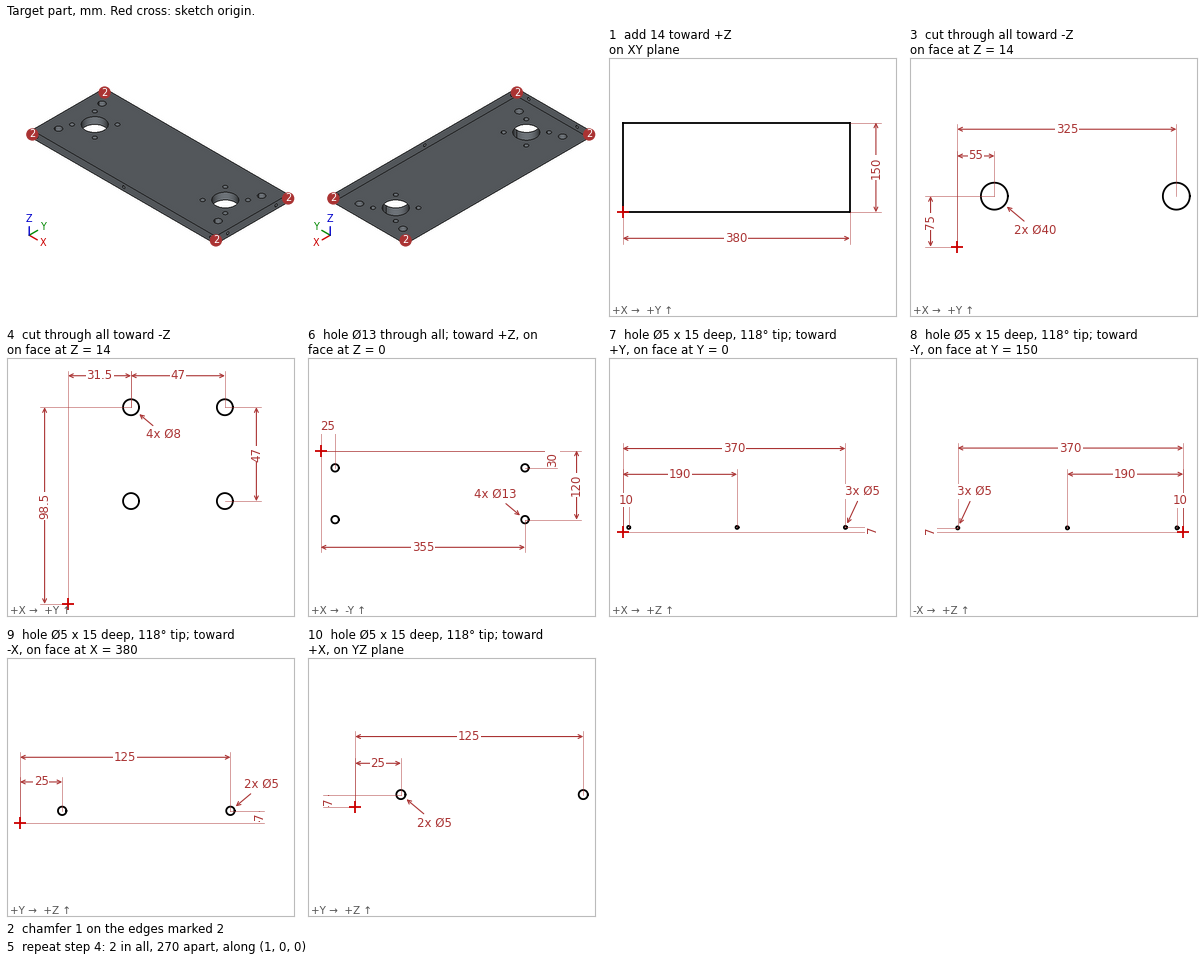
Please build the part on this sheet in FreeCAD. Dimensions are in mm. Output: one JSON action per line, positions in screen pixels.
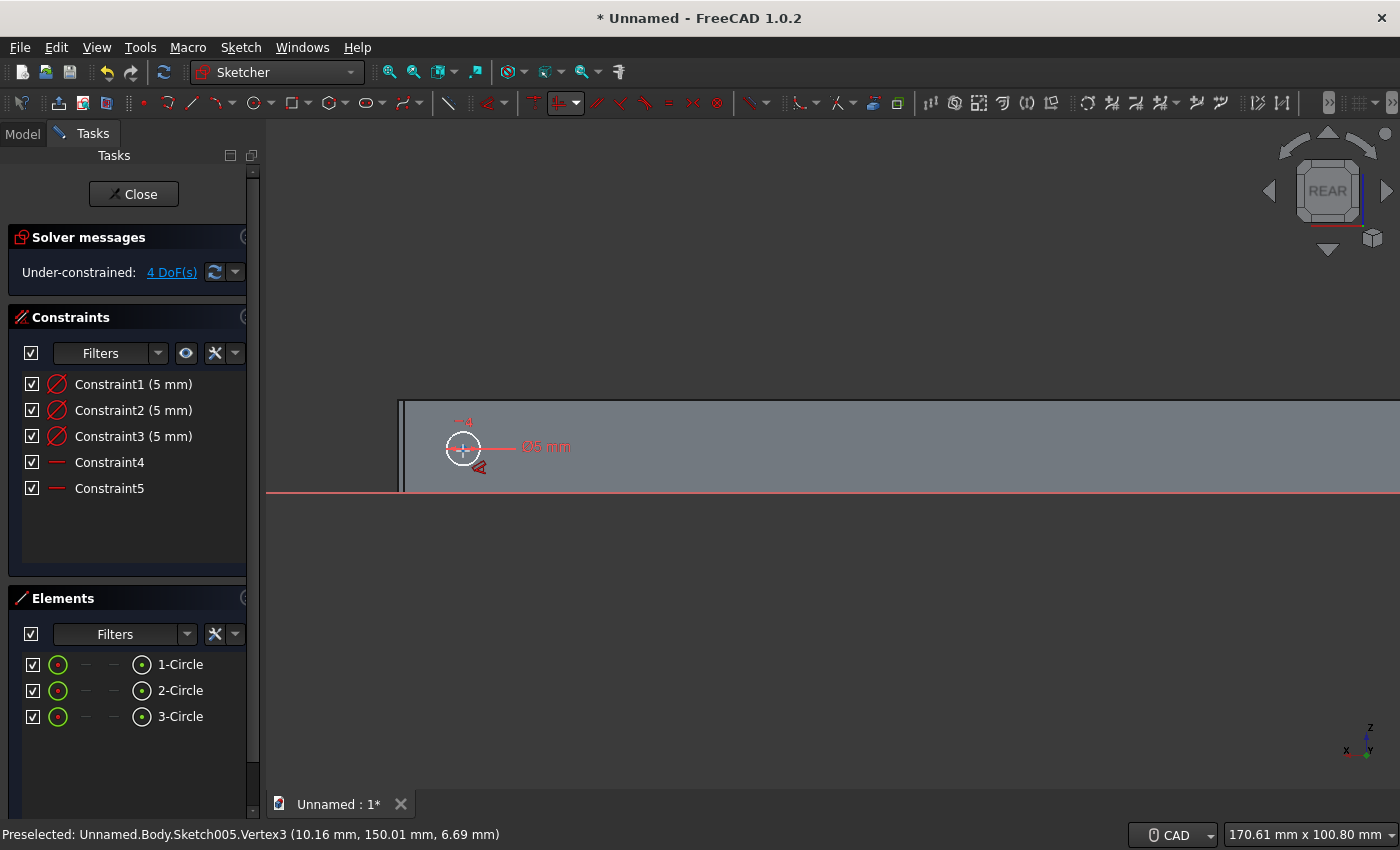
{"action": "left_click", "coordinate": [463, 449]}
{"action": "left_click", "coordinate": [429, 471]}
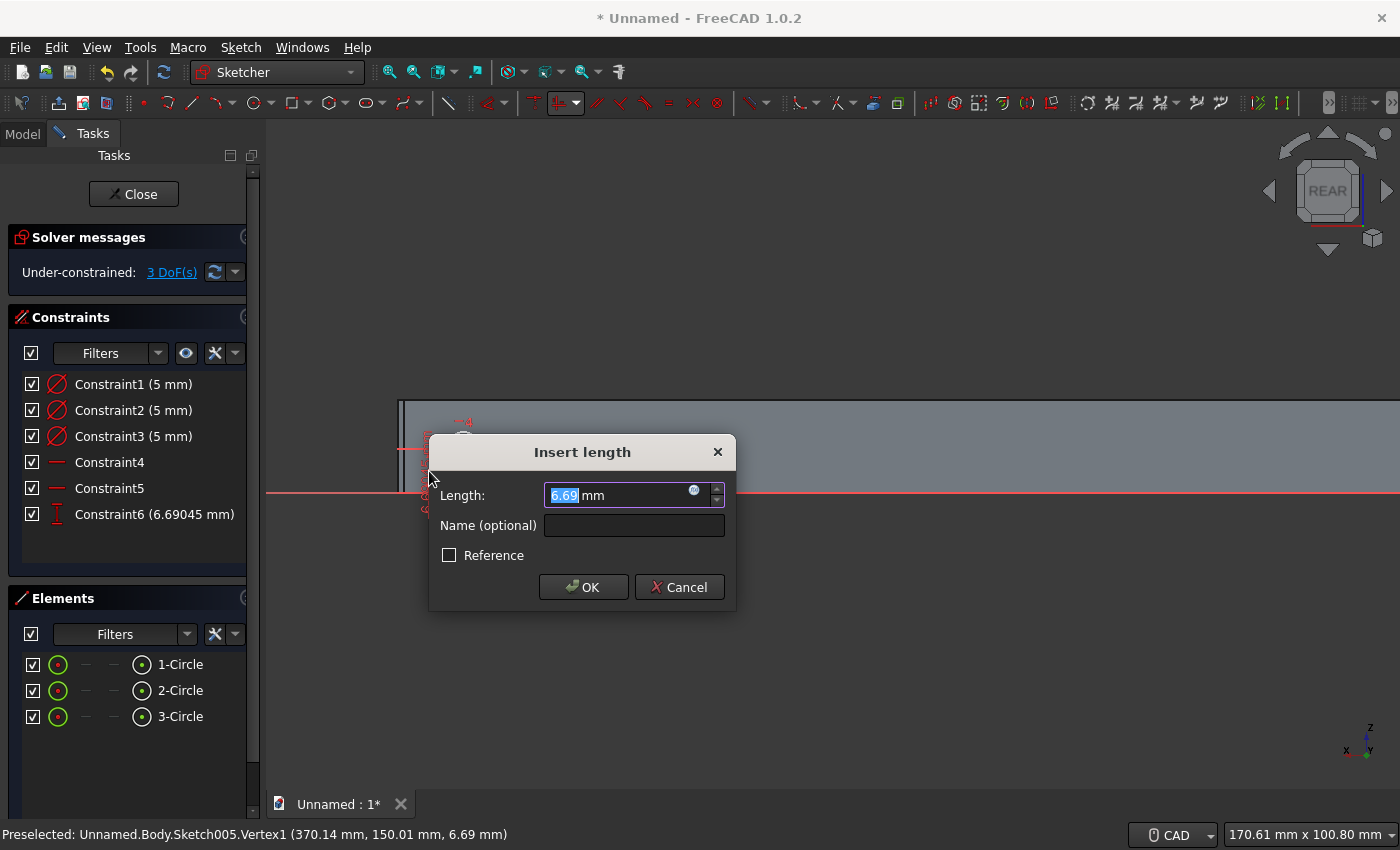
{"action": "type", "text": "7"}
{"action": "key", "text": "Return"}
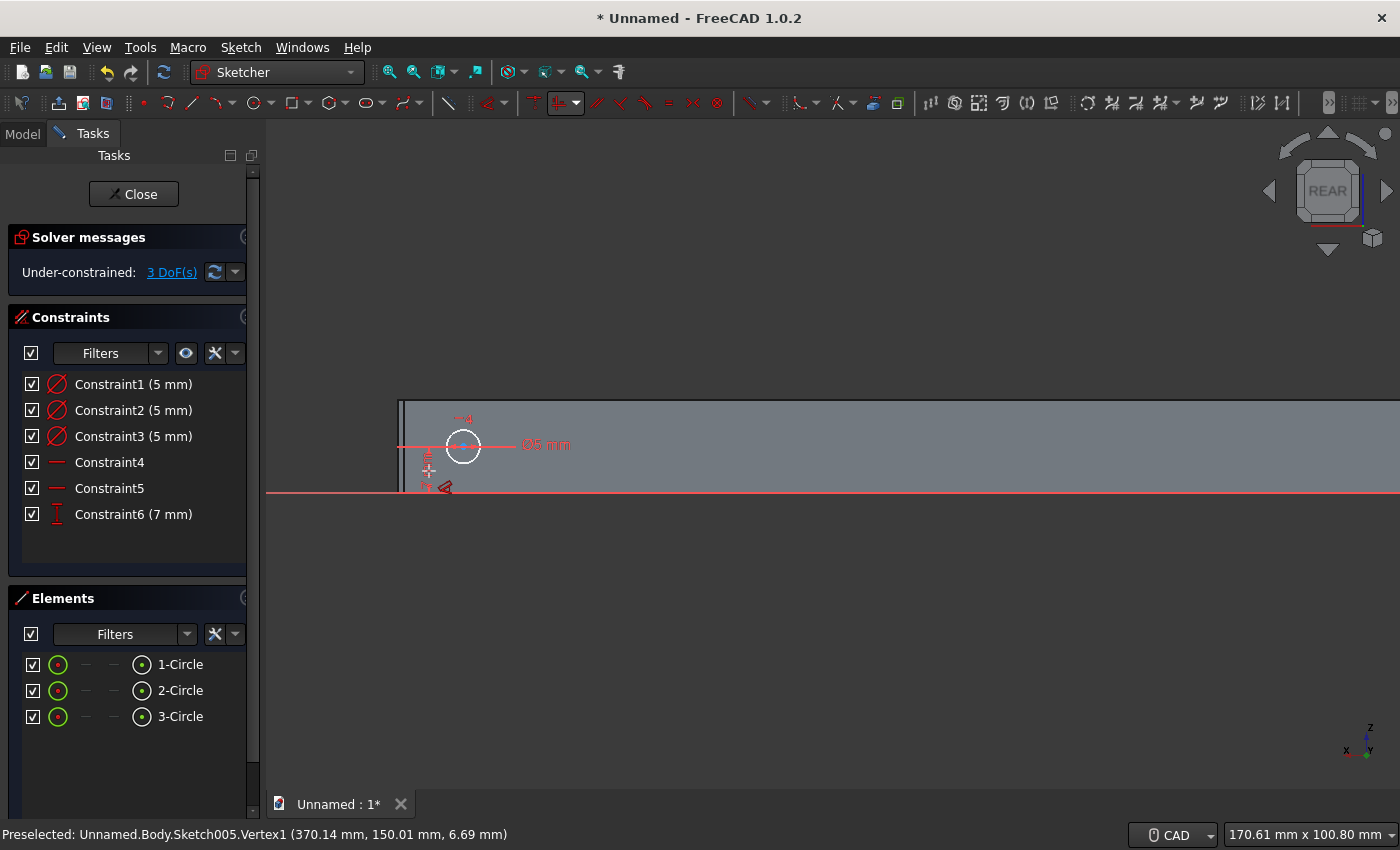
{"action": "scroll", "coordinate": [463, 451], "scroll_direction": "down", "scroll_amount": 7}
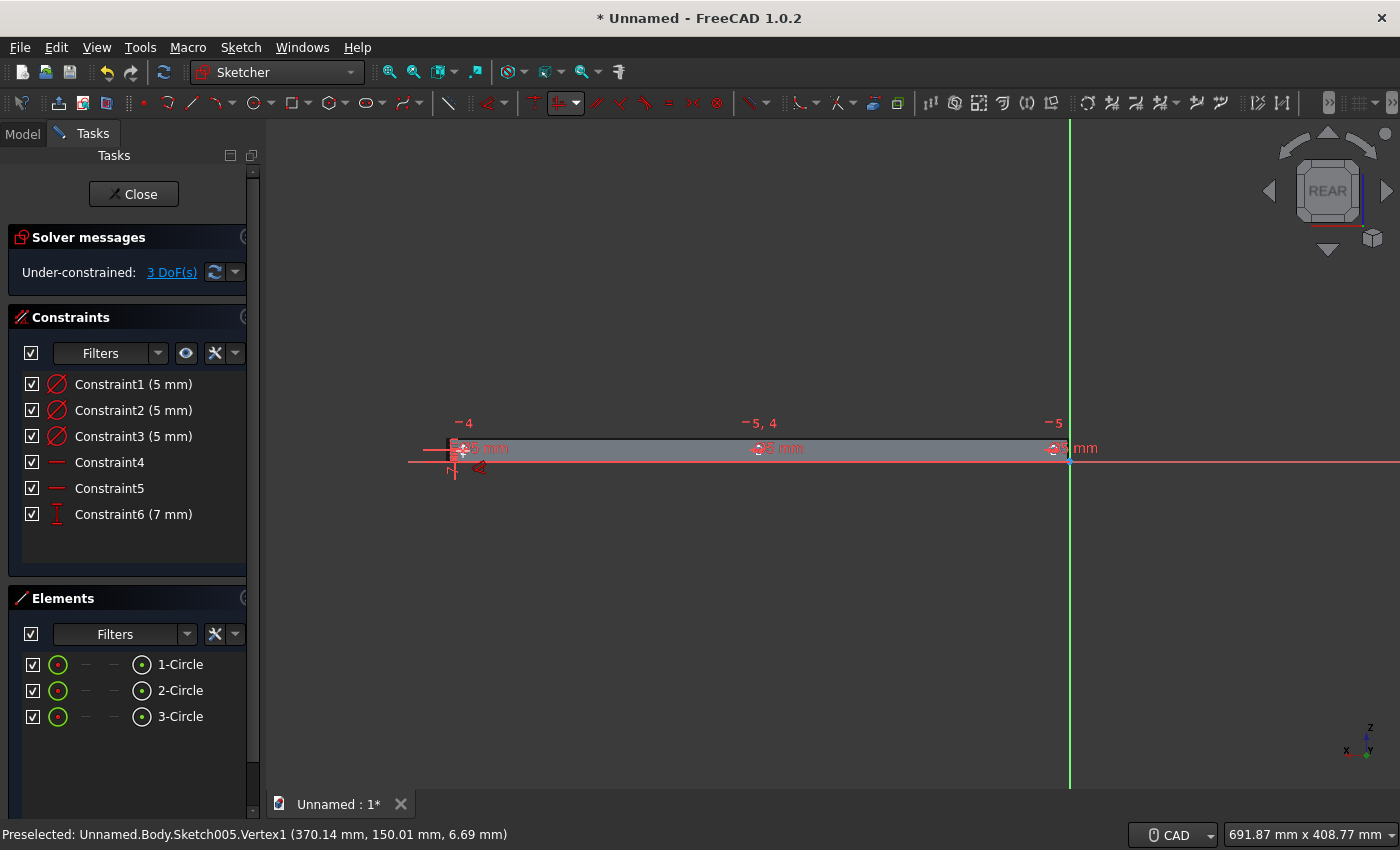
{"action": "scroll", "coordinate": [1053, 450], "scroll_direction": "up", "scroll_amount": 5}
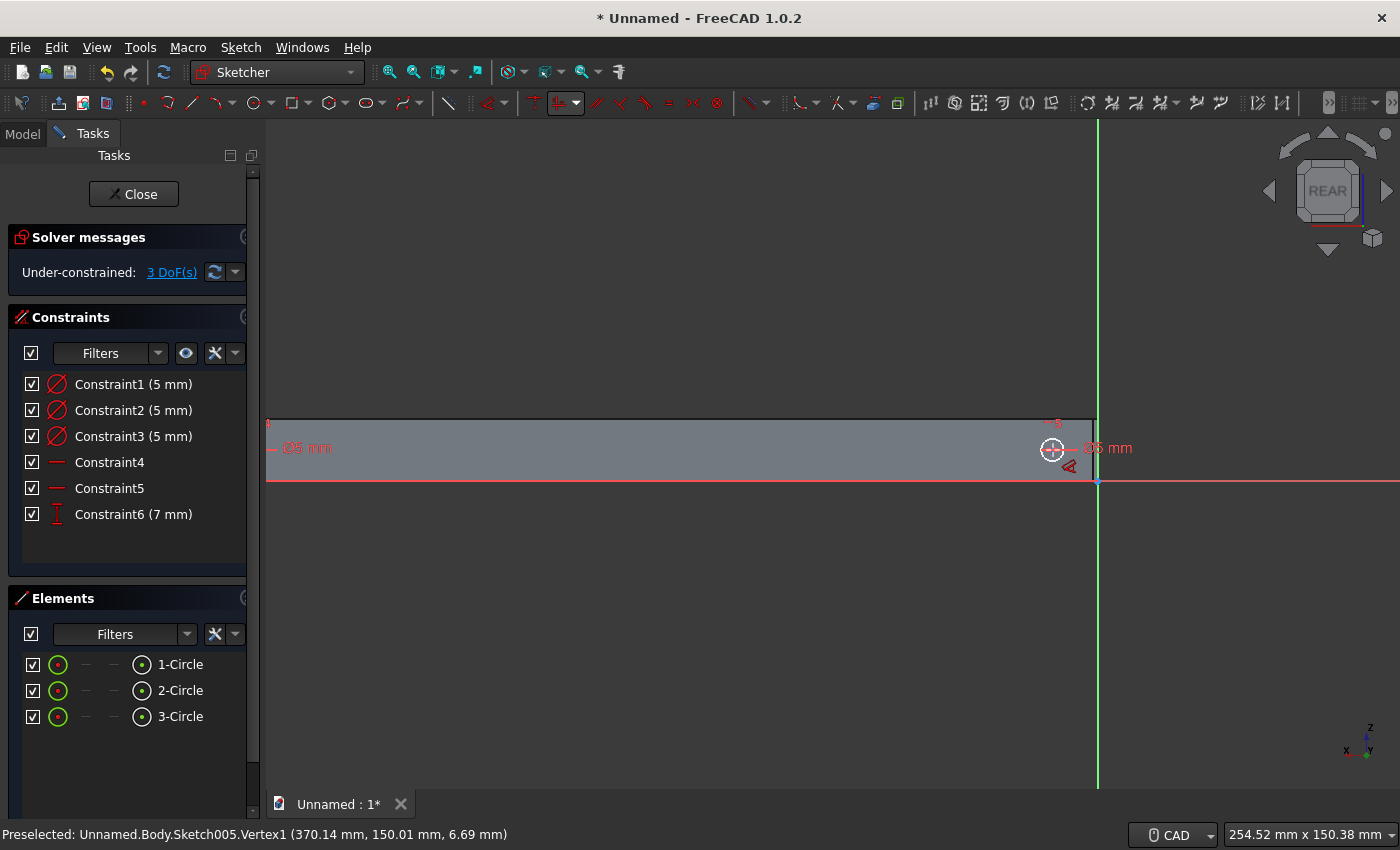
{"action": "left_click", "coordinate": [1052, 450]}
{"action": "left_click", "coordinate": [1075, 515]}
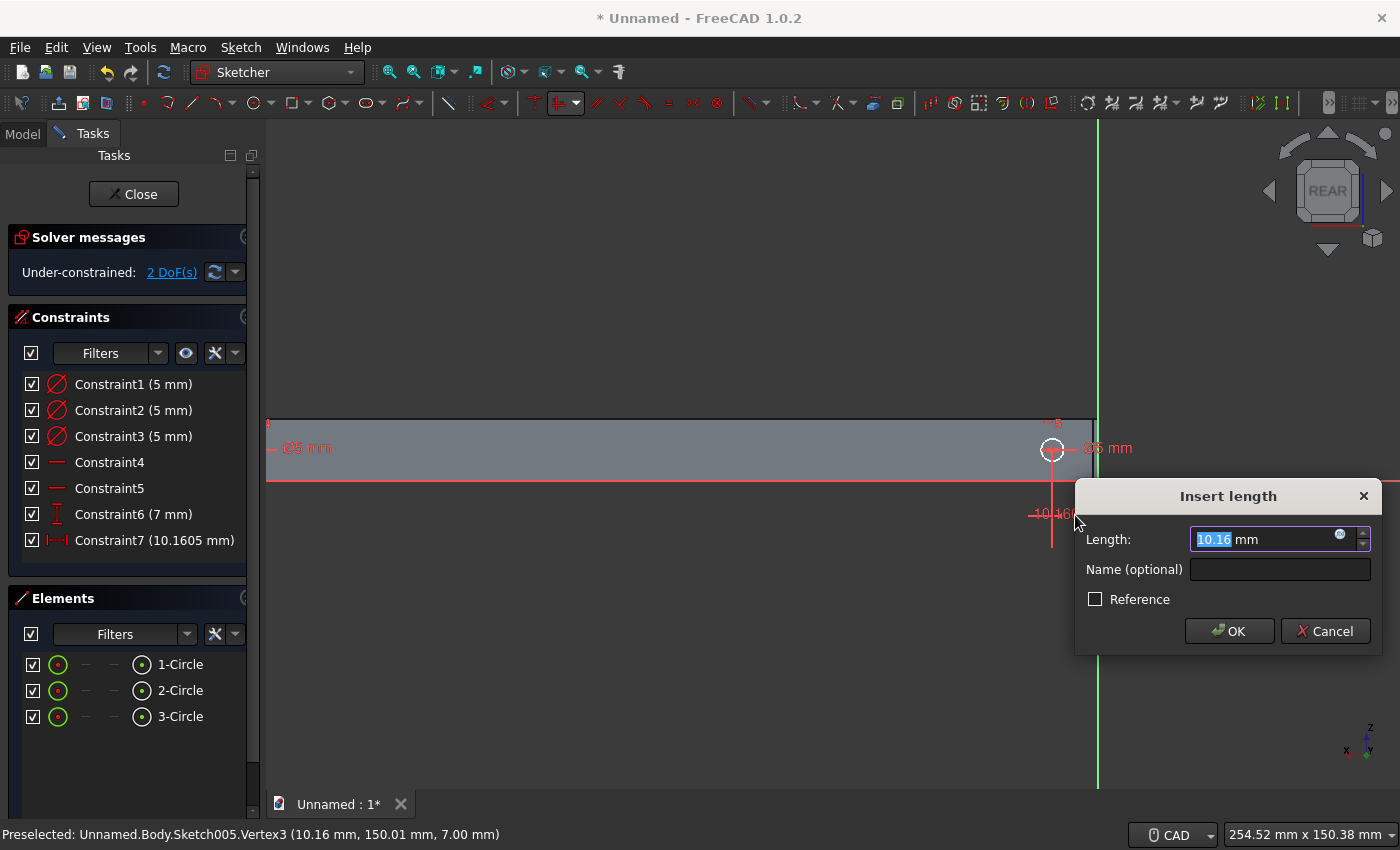
{"action": "type", "text": "10"}
{"action": "key", "text": "Return"}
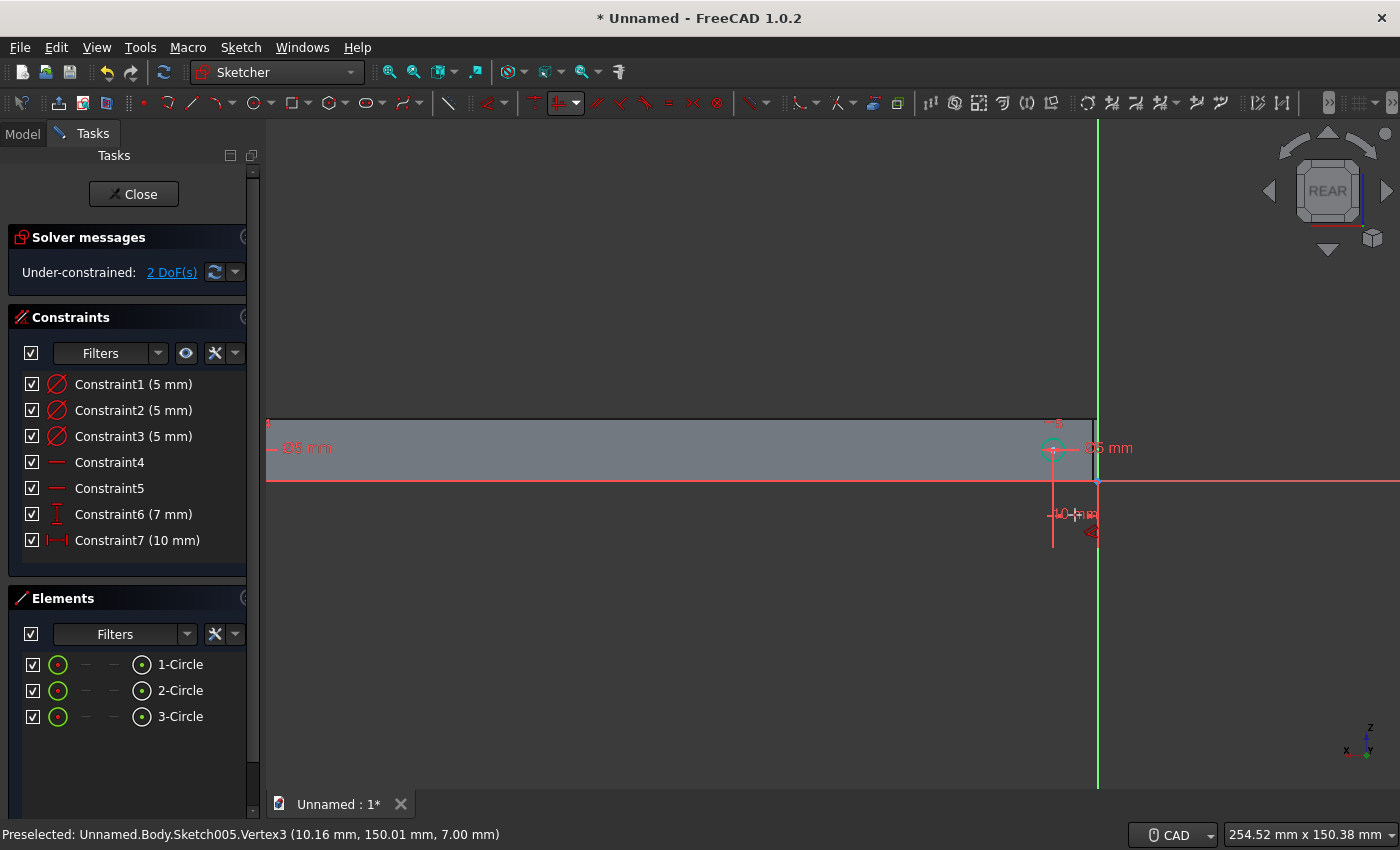
{"action": "scroll", "coordinate": [1054, 450], "scroll_direction": "down", "scroll_amount": 5}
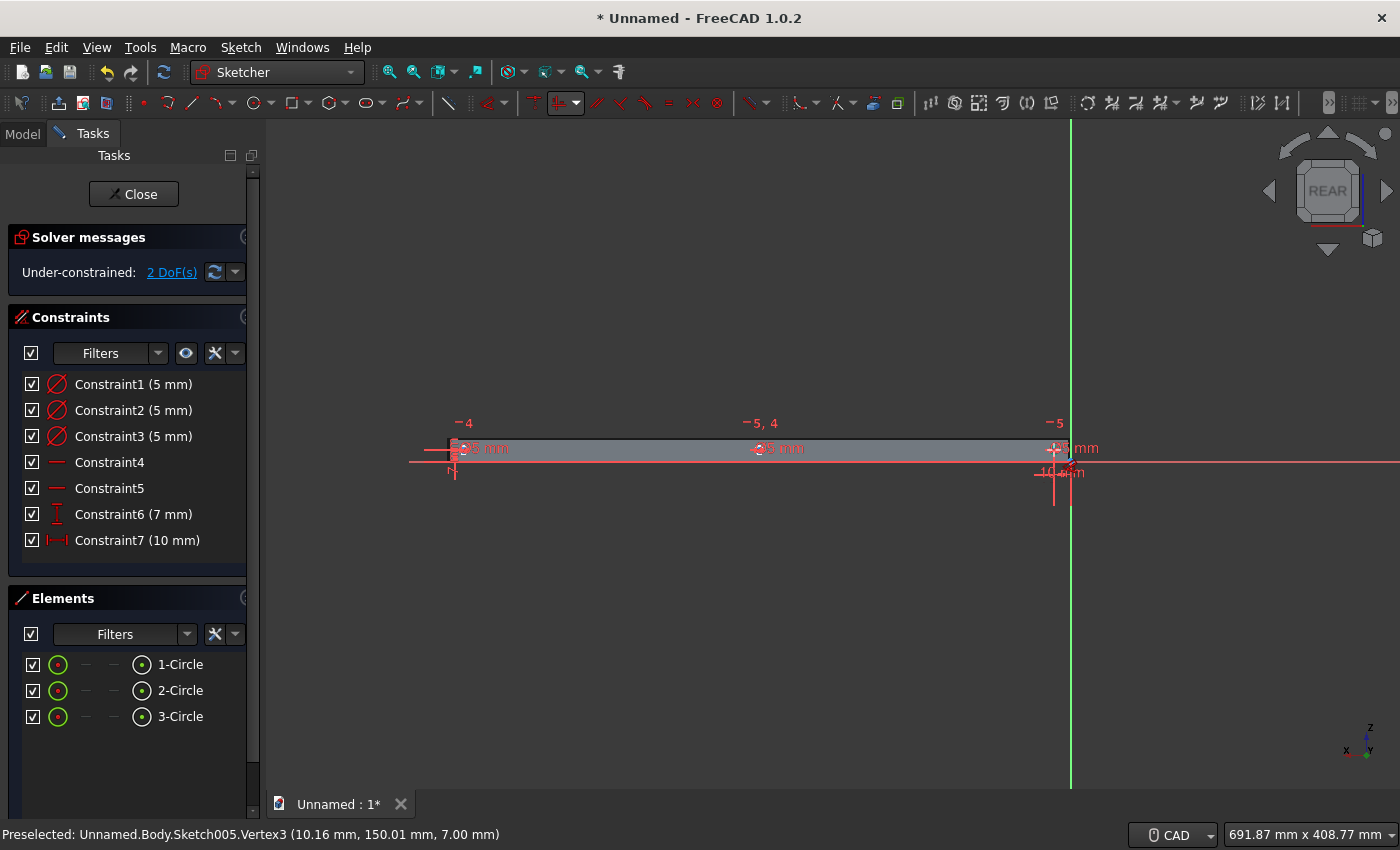
{"action": "left_click", "coordinate": [464, 450]}
{"action": "left_click", "coordinate": [767, 496]}